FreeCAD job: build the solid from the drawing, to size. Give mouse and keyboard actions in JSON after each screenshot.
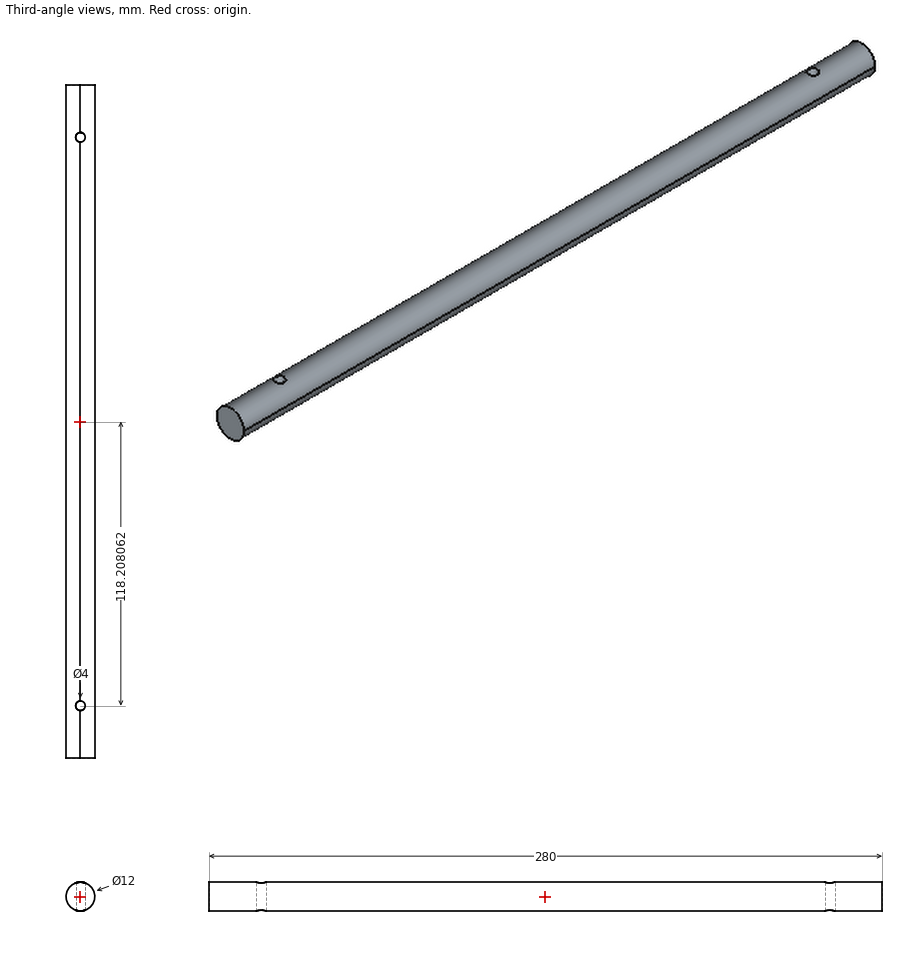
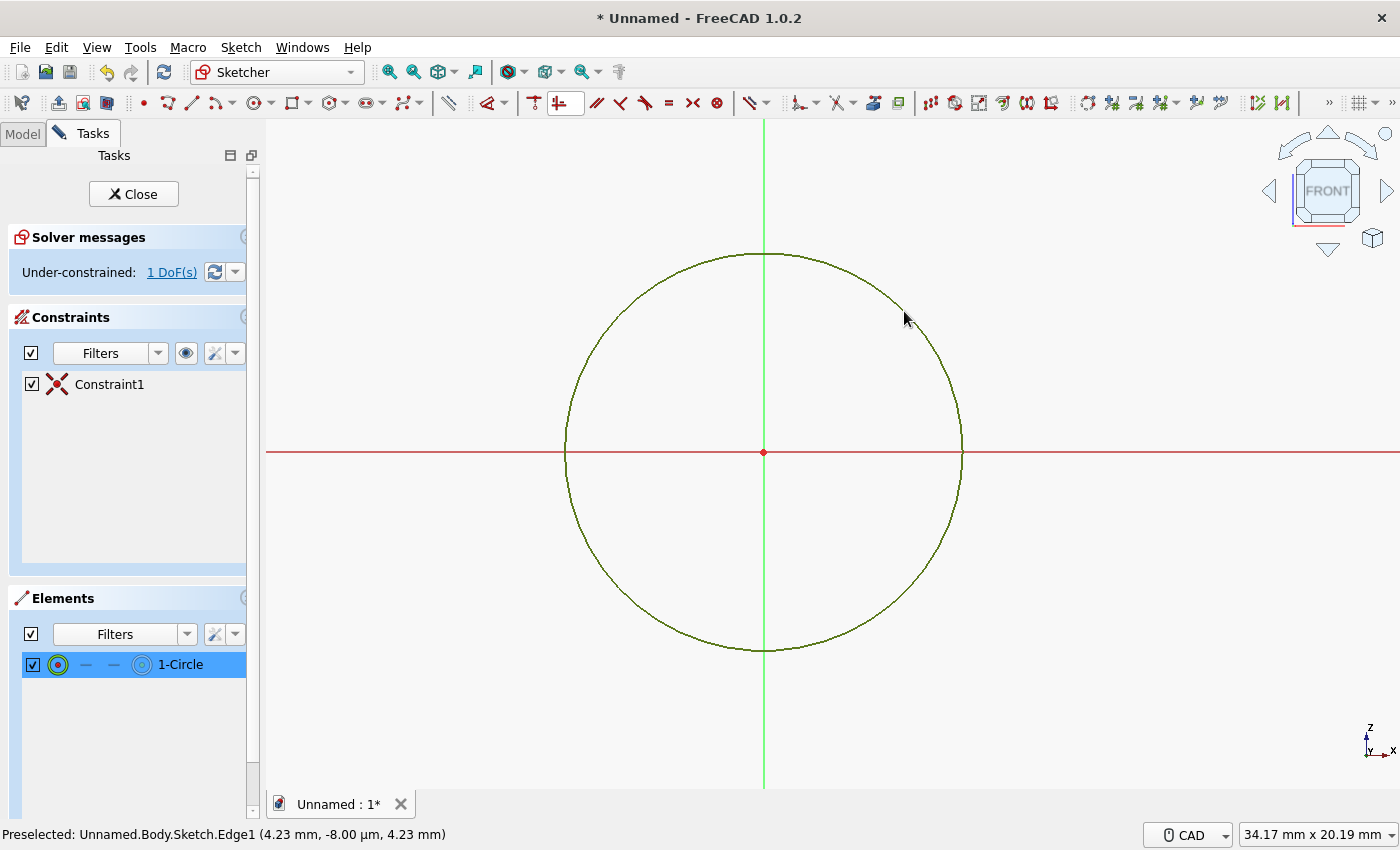
{"action": "key", "text": "k o"}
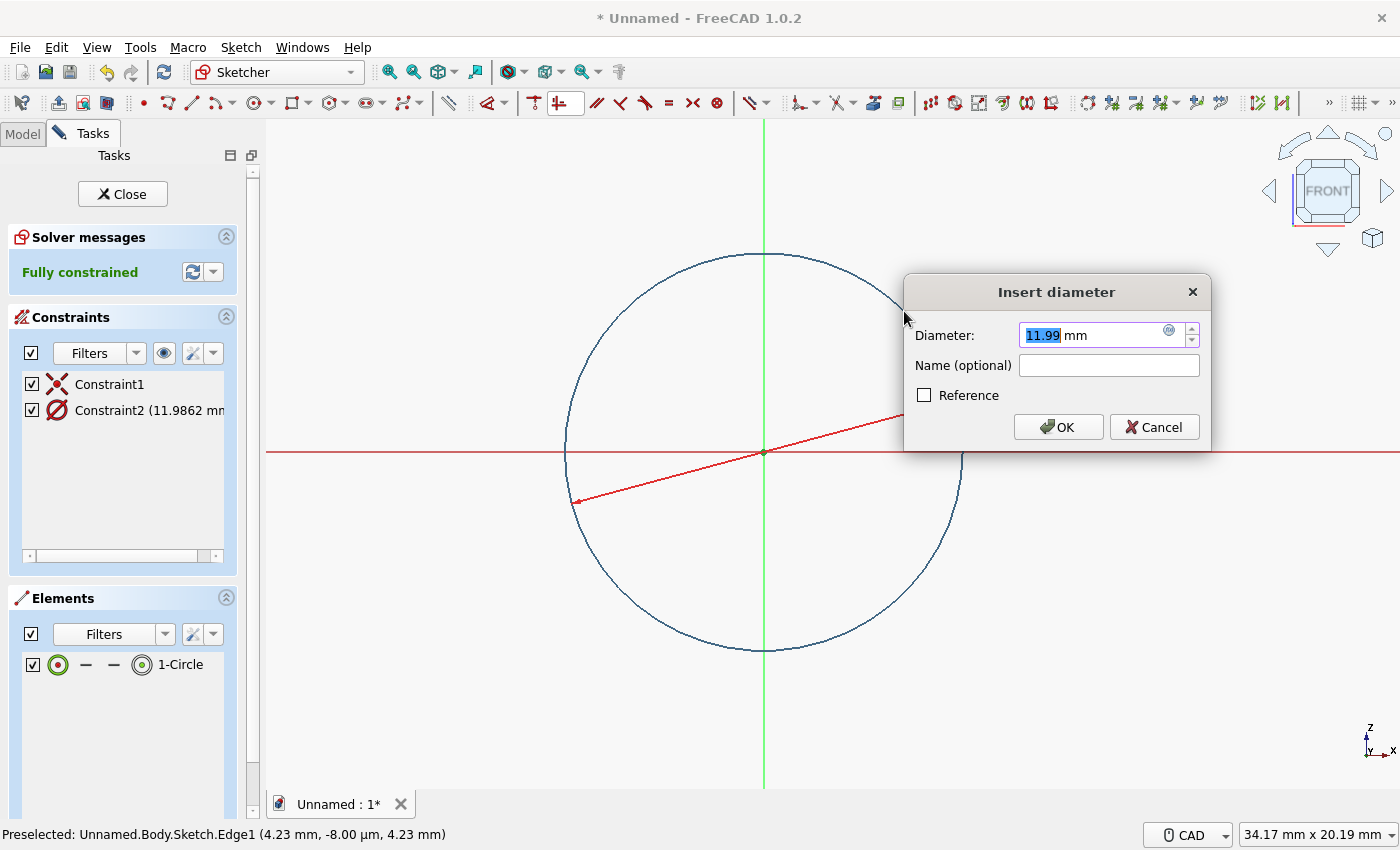
{"action": "type", "text": "12"}
{"action": "key", "text": "Return"}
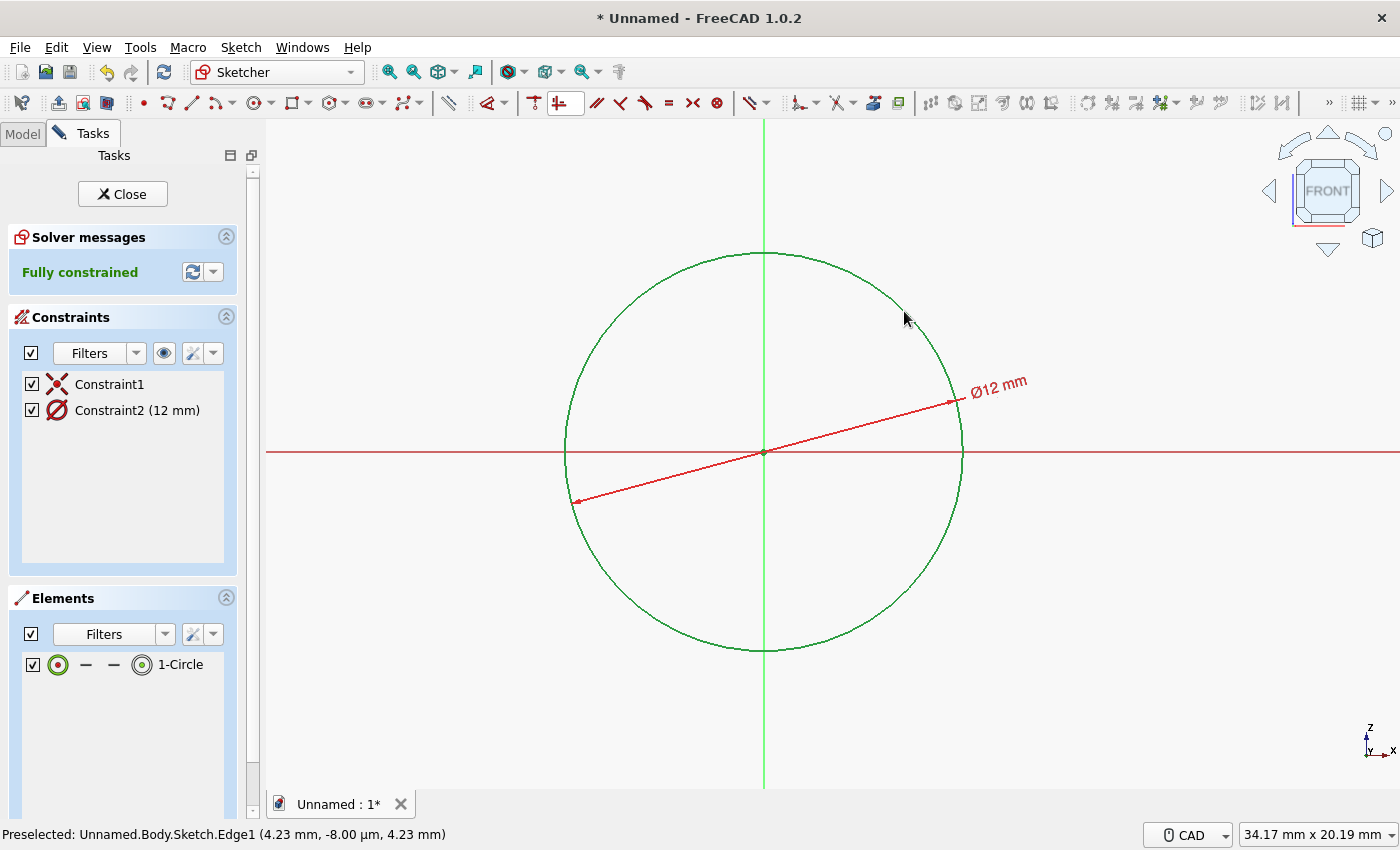
{"action": "left_click", "coordinate": [123, 194]}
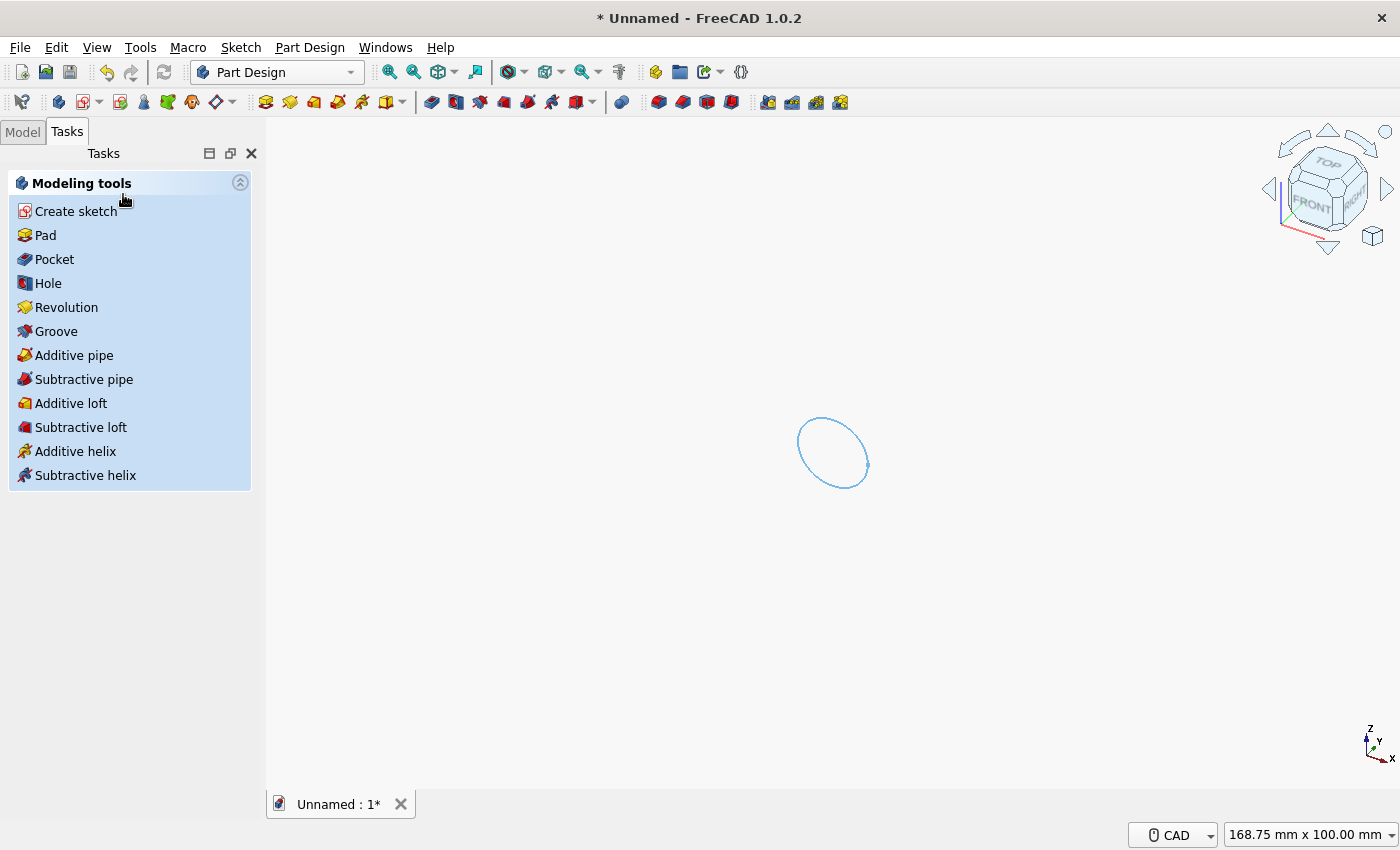
{"action": "left_click", "coordinate": [266, 102]}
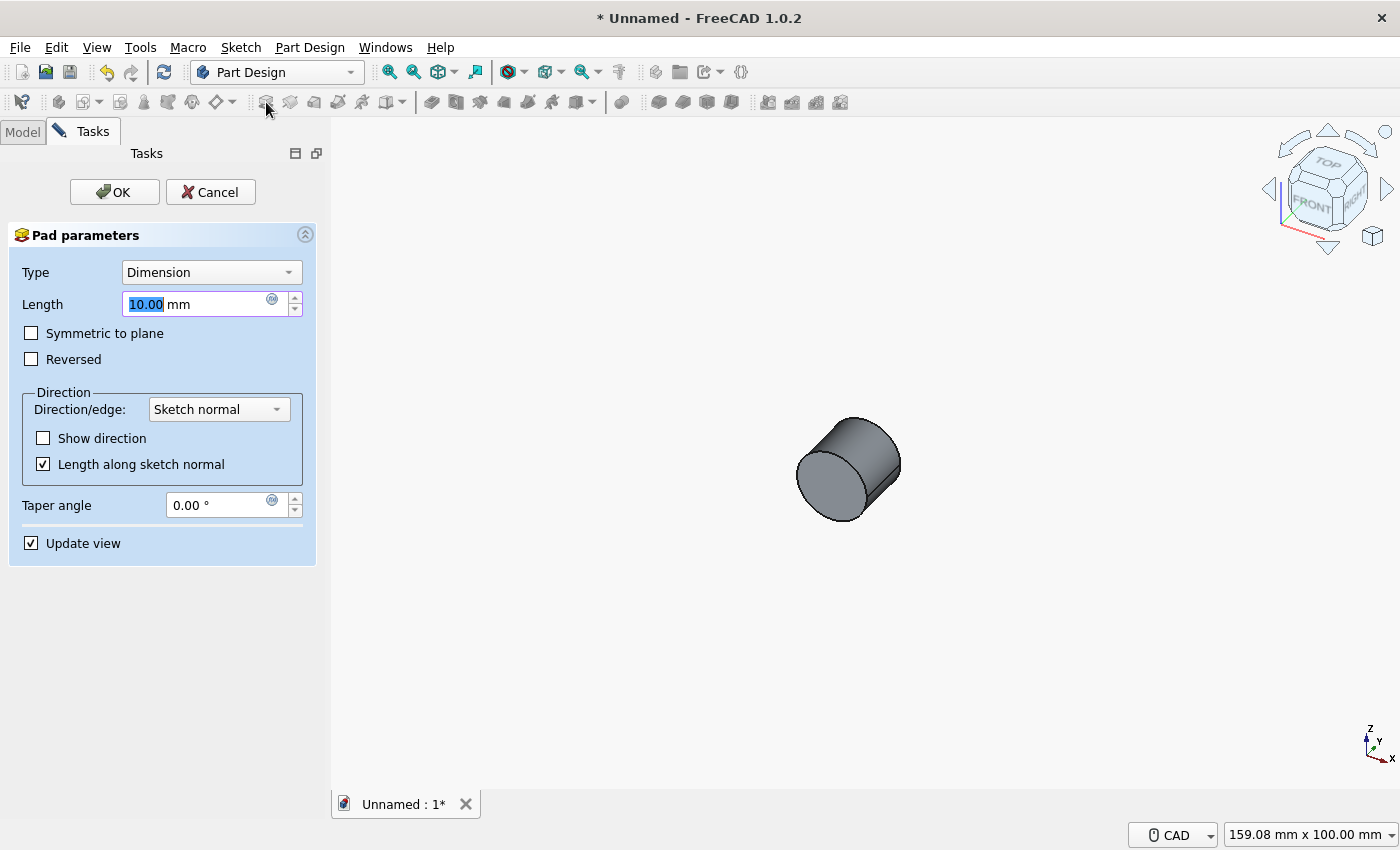
{"action": "type", "text": "280"}
{"action": "key", "text": "Tab"}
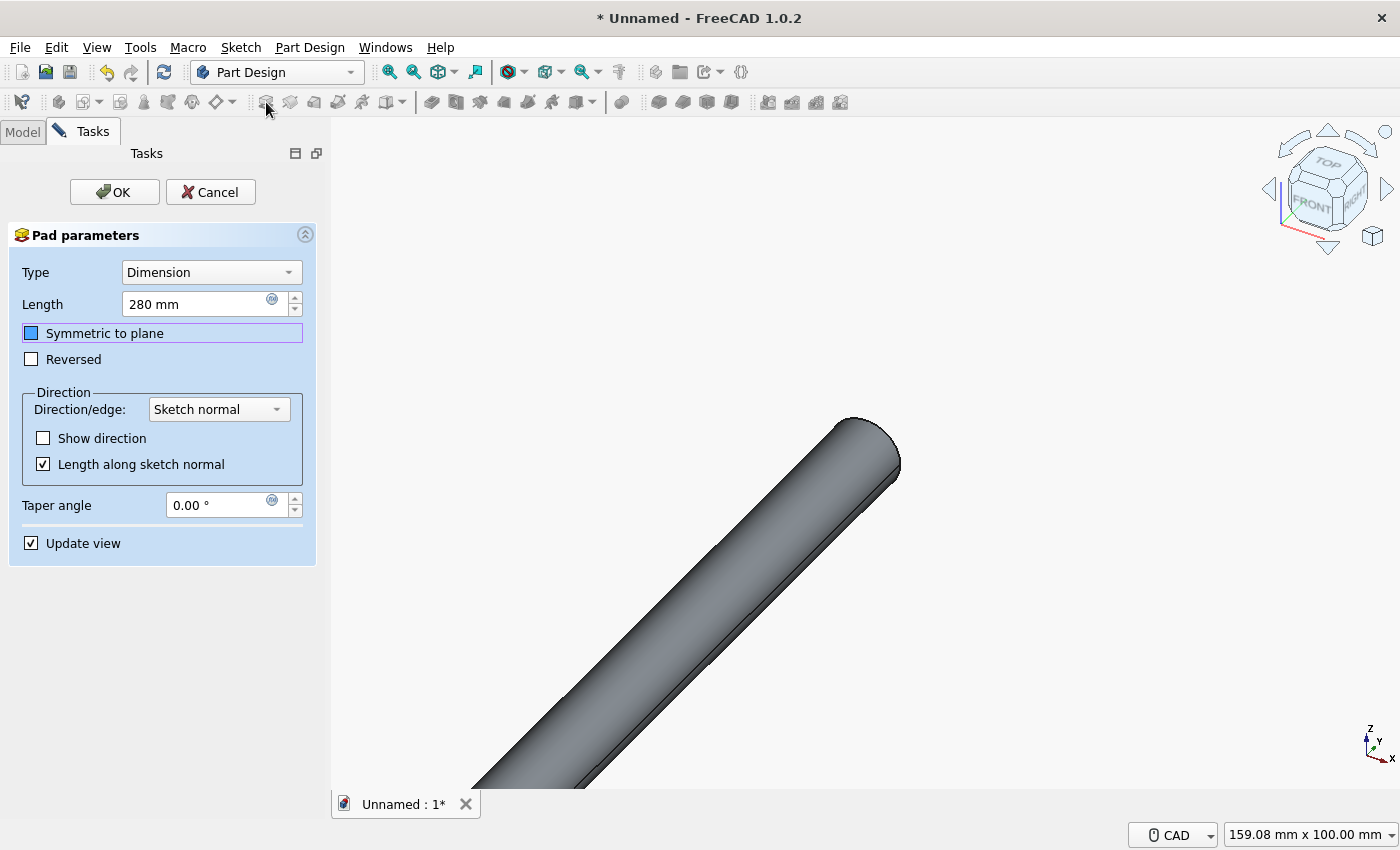
{"action": "left_click", "coordinate": [30, 333]}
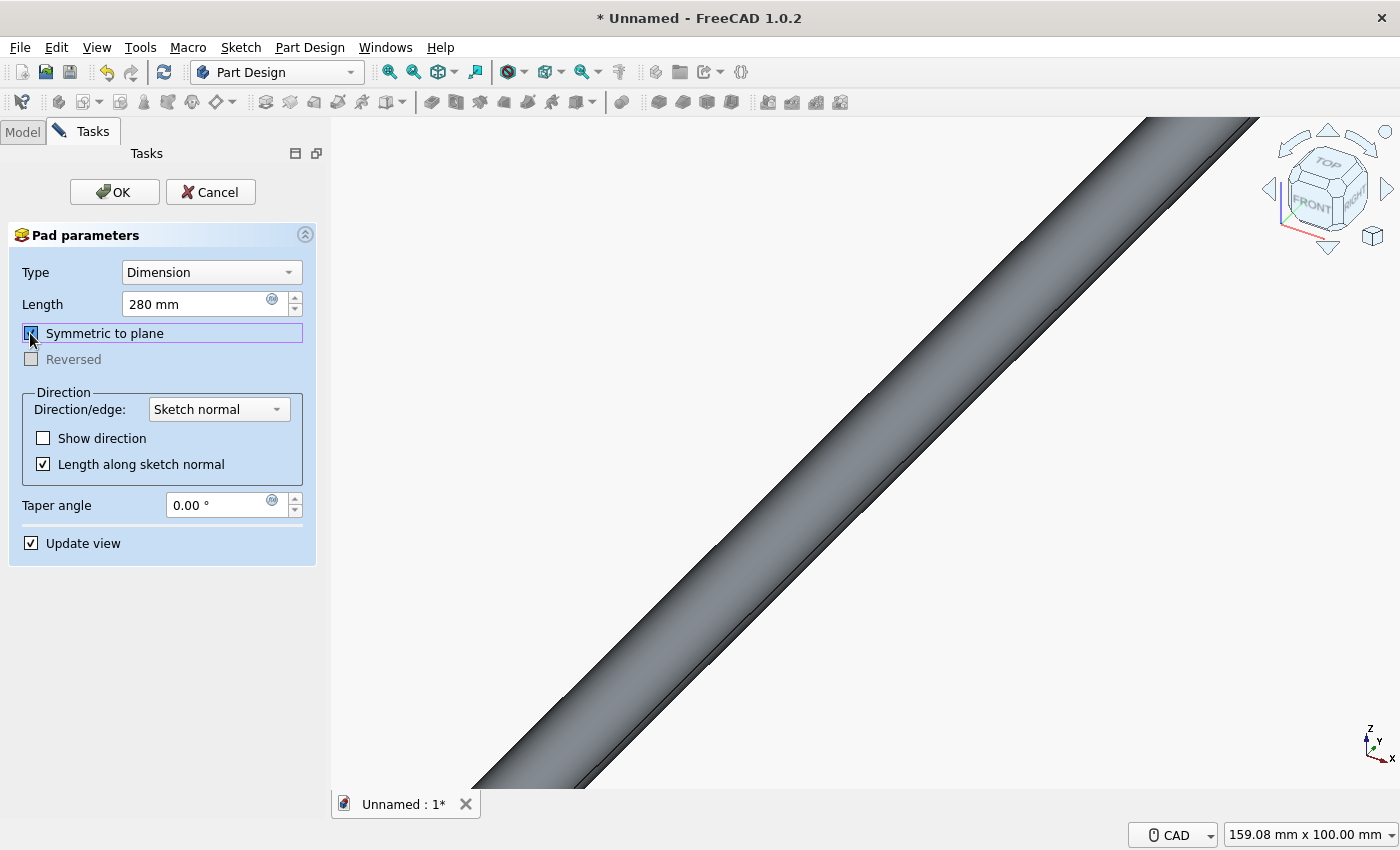
{"action": "left_click", "coordinate": [115, 192]}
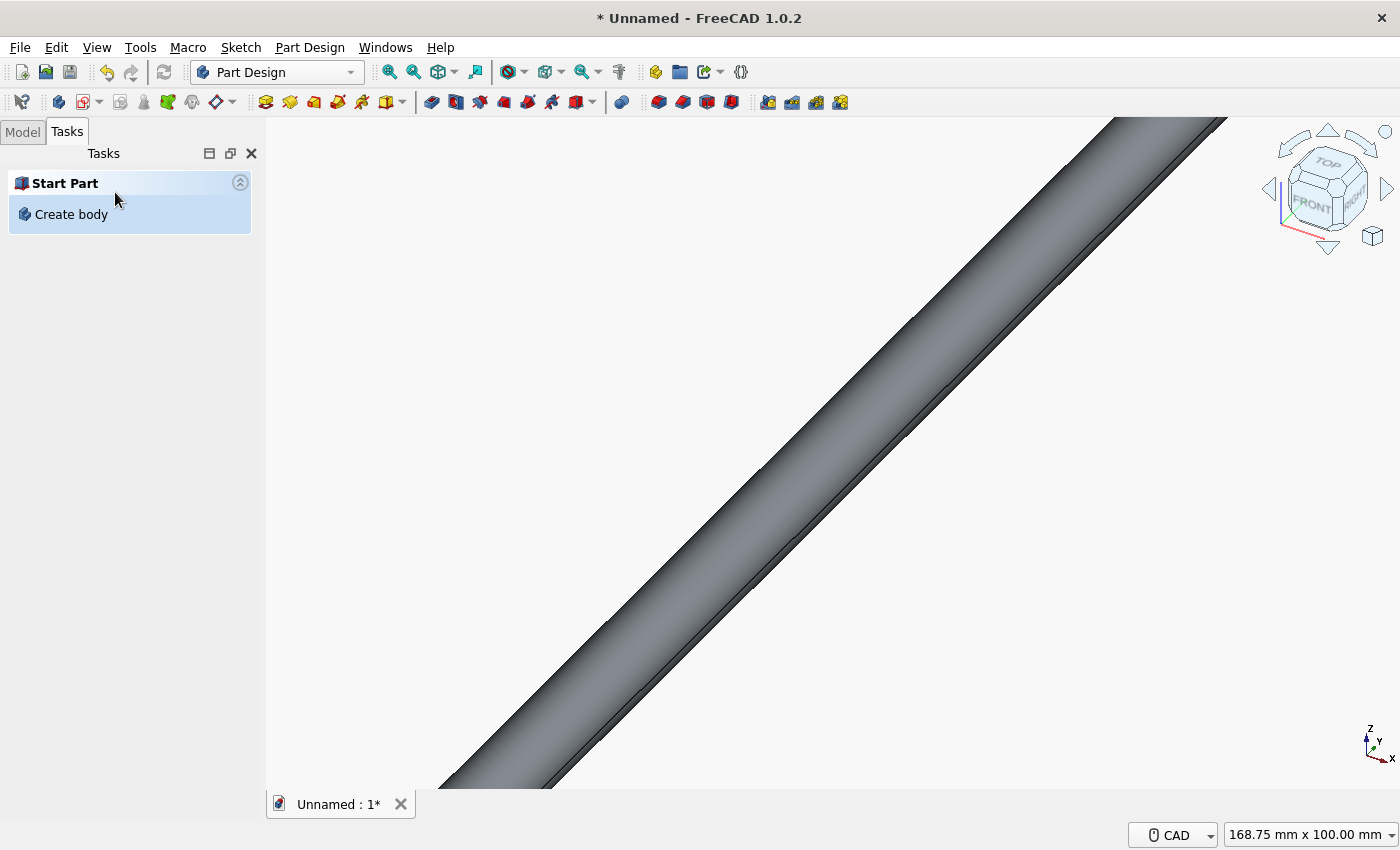
{"action": "left_click", "coordinate": [390, 72]}